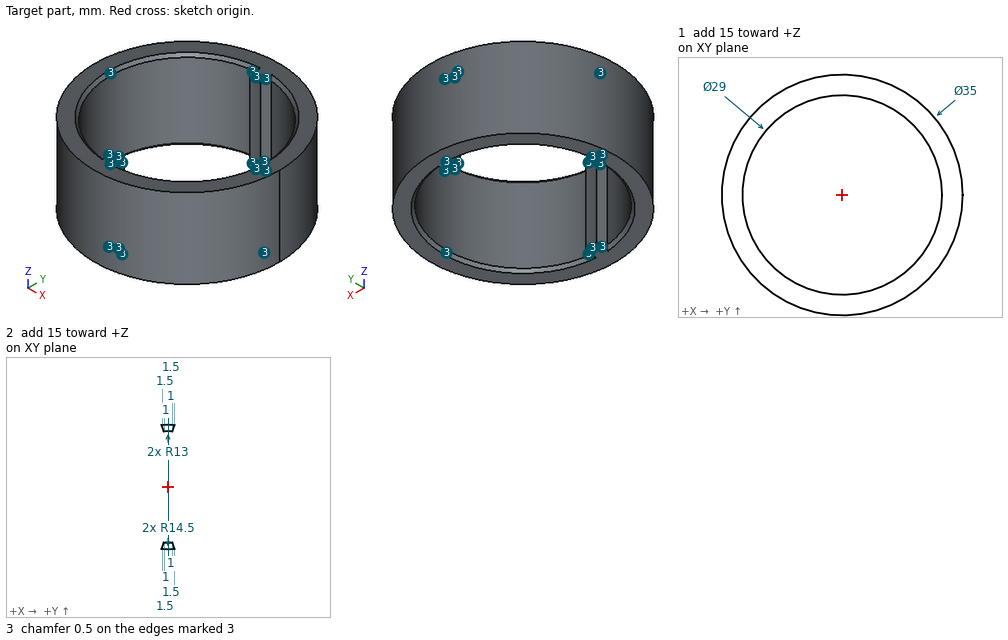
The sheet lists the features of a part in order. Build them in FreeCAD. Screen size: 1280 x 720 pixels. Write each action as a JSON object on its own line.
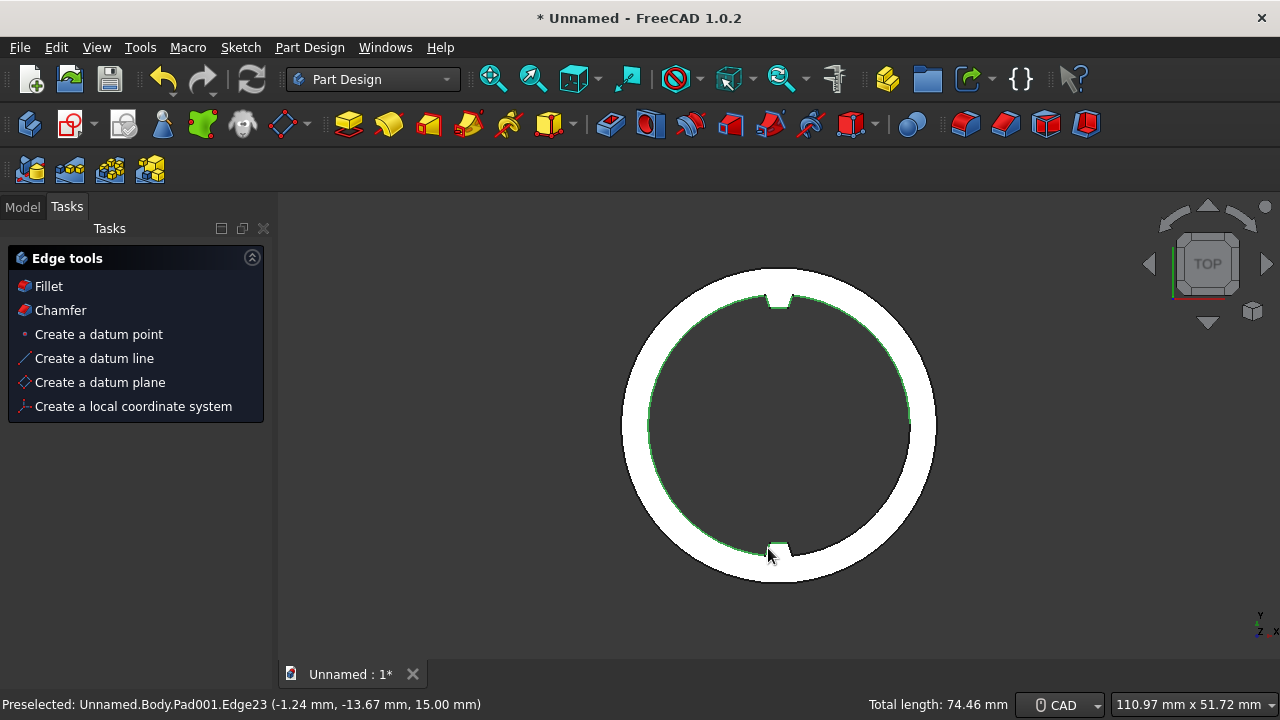
{"action": "left_click", "coordinate": [790, 548], "text": "ctrl"}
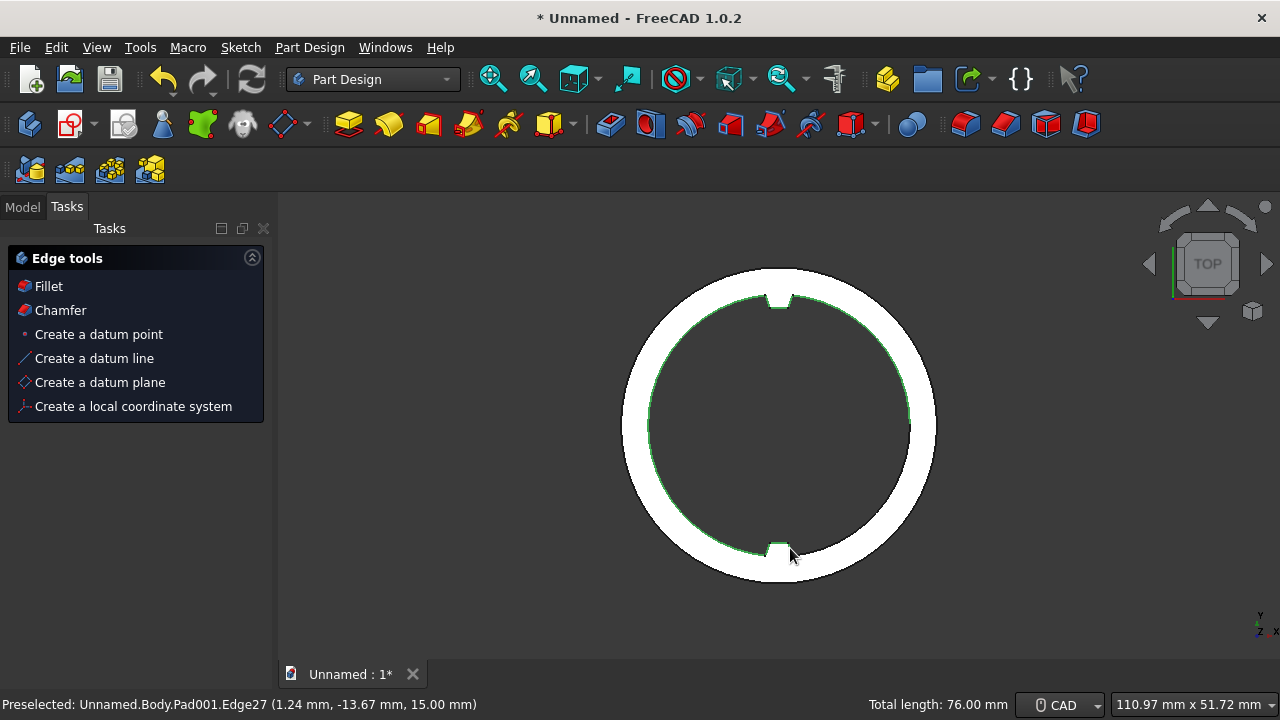
{"action": "key", "text": "1"}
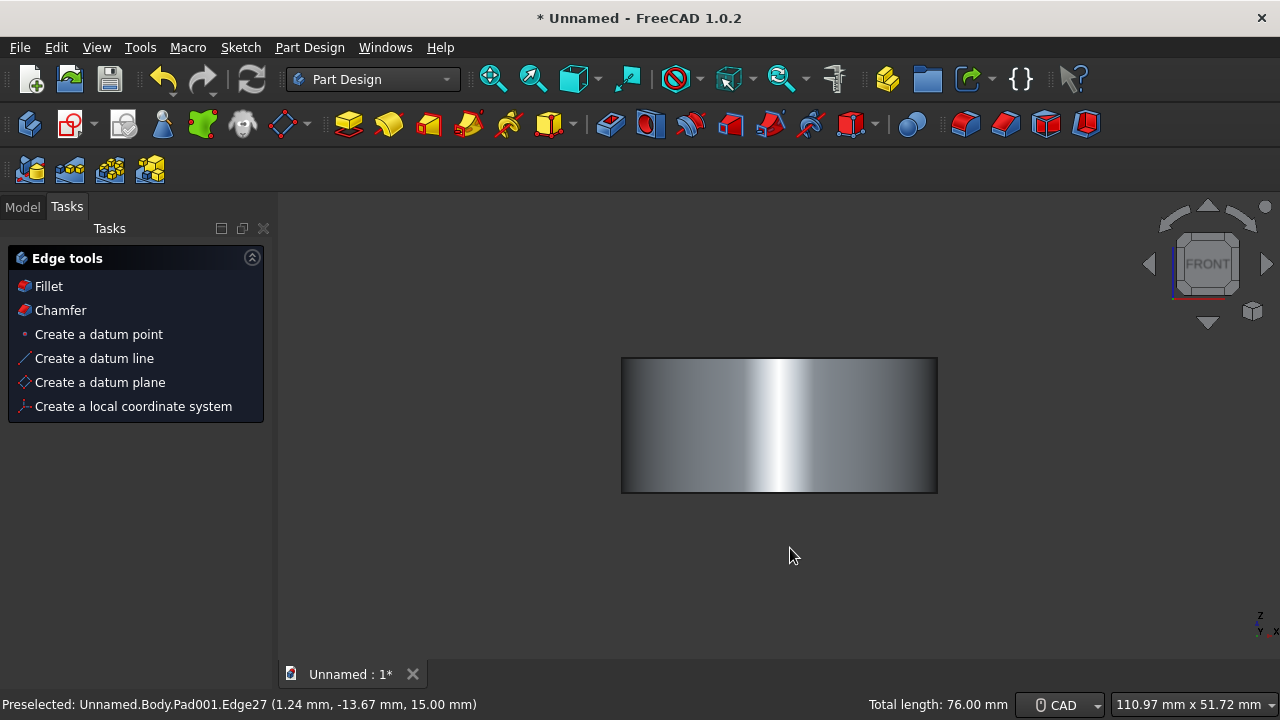
{"action": "left_click", "coordinate": [494, 80]}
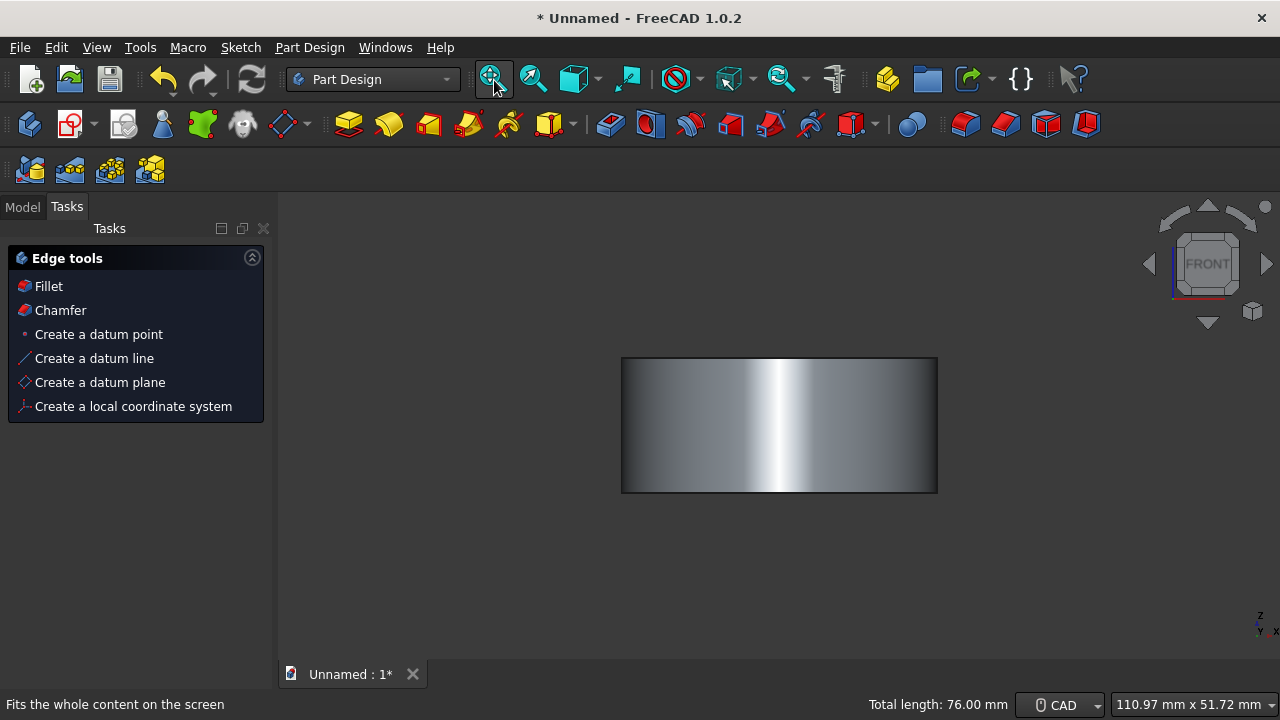
{"action": "key", "text": "3"}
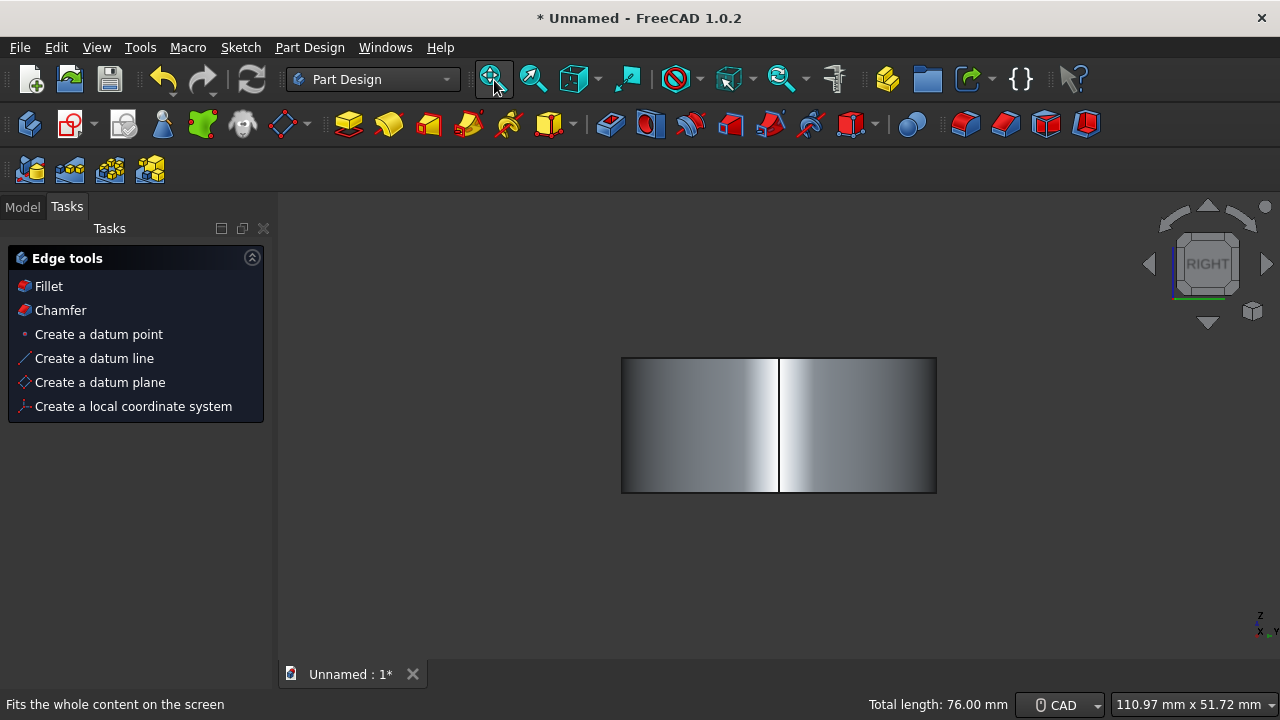
{"action": "left_click", "coordinate": [494, 80]}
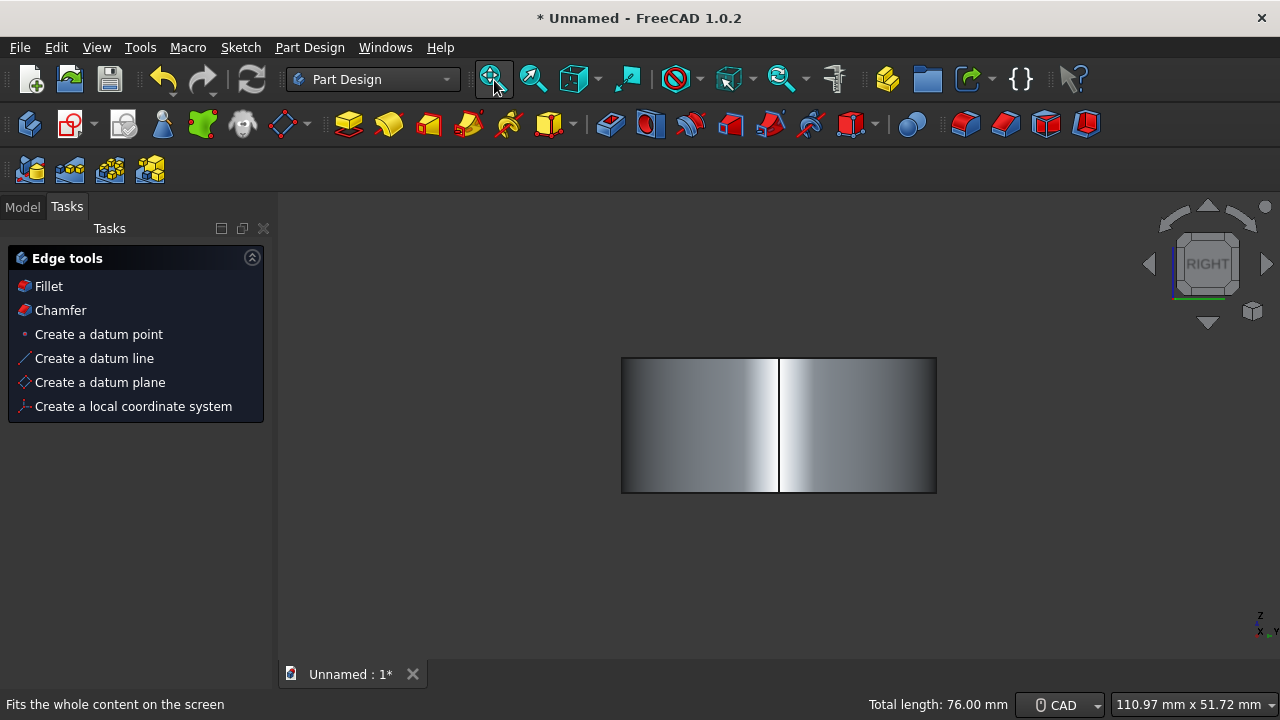
{"action": "key", "text": "5"}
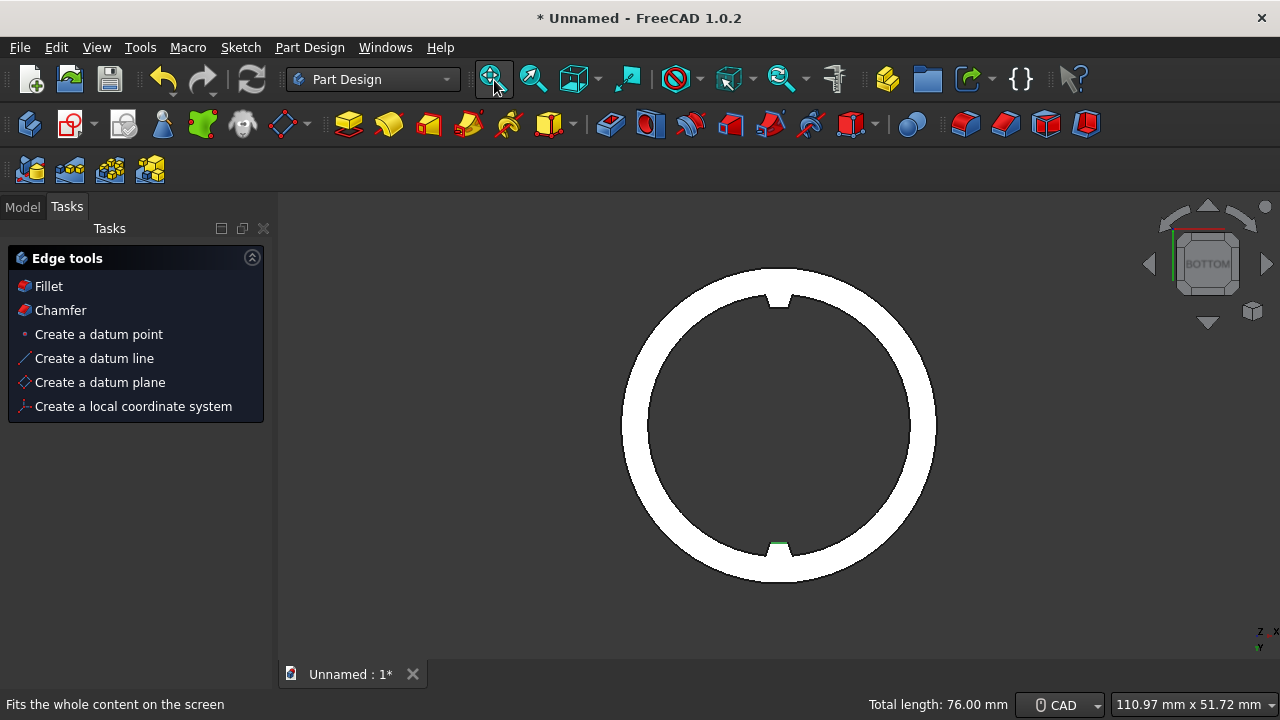
{"action": "left_click", "coordinate": [648, 424], "text": "ctrl"}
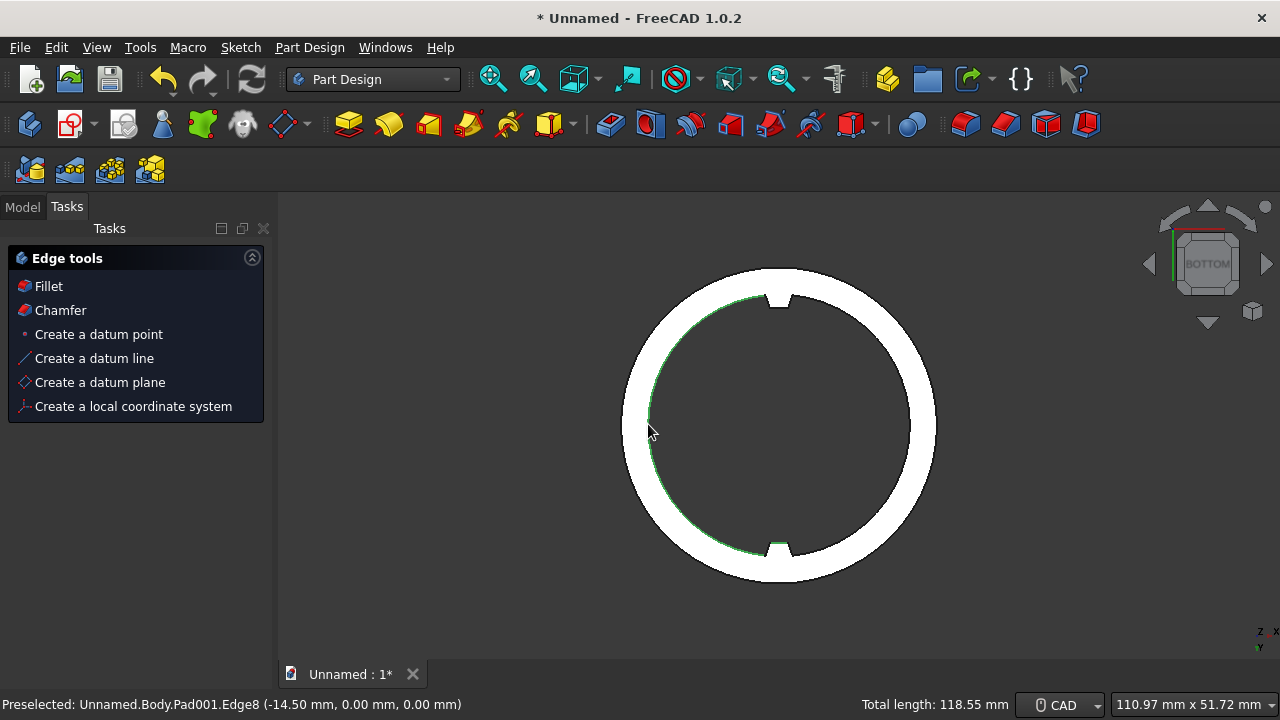
{"action": "left_click", "coordinate": [768, 548], "text": "ctrl"}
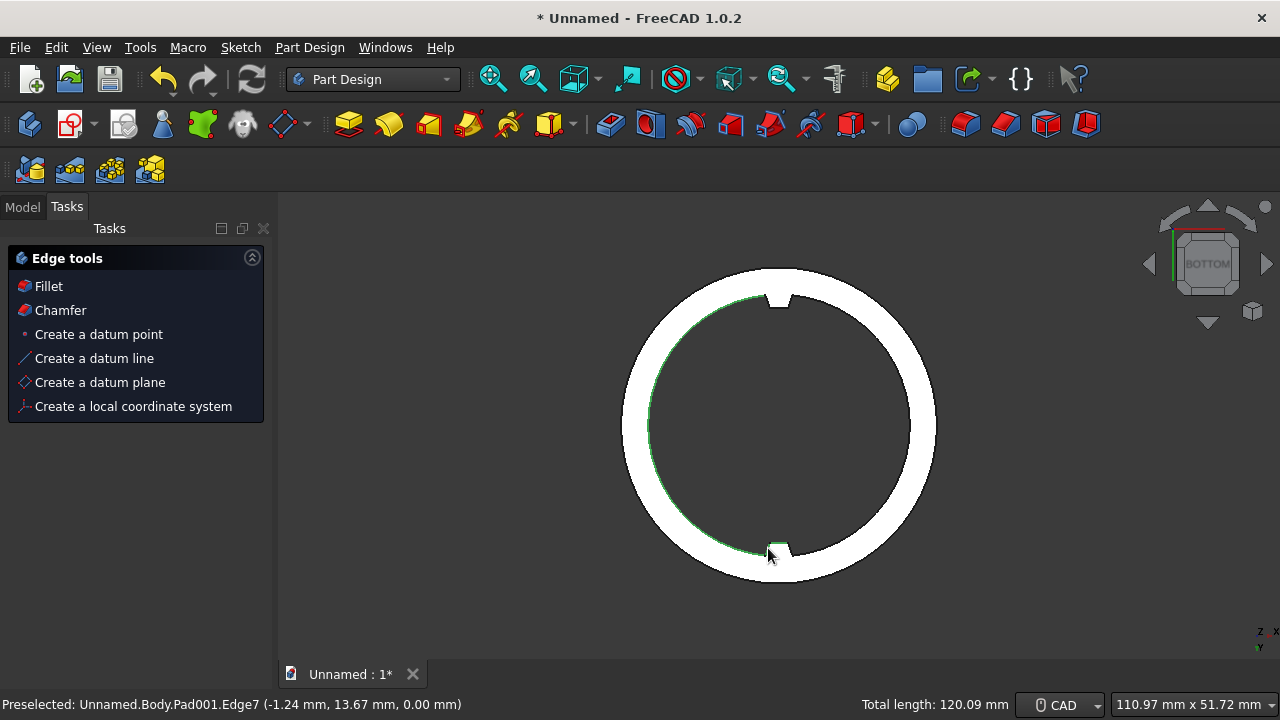
{"action": "left_click", "coordinate": [790, 548], "text": "ctrl"}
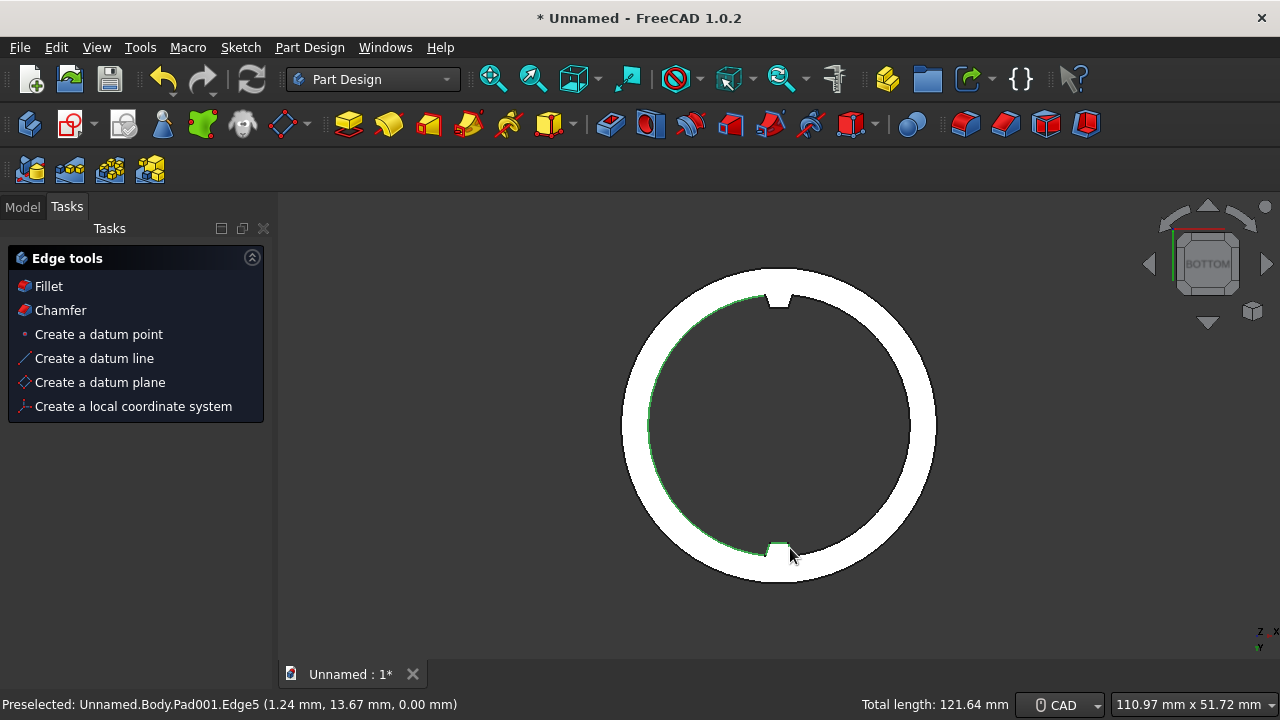
{"action": "left_click", "coordinate": [862, 525], "text": "ctrl"}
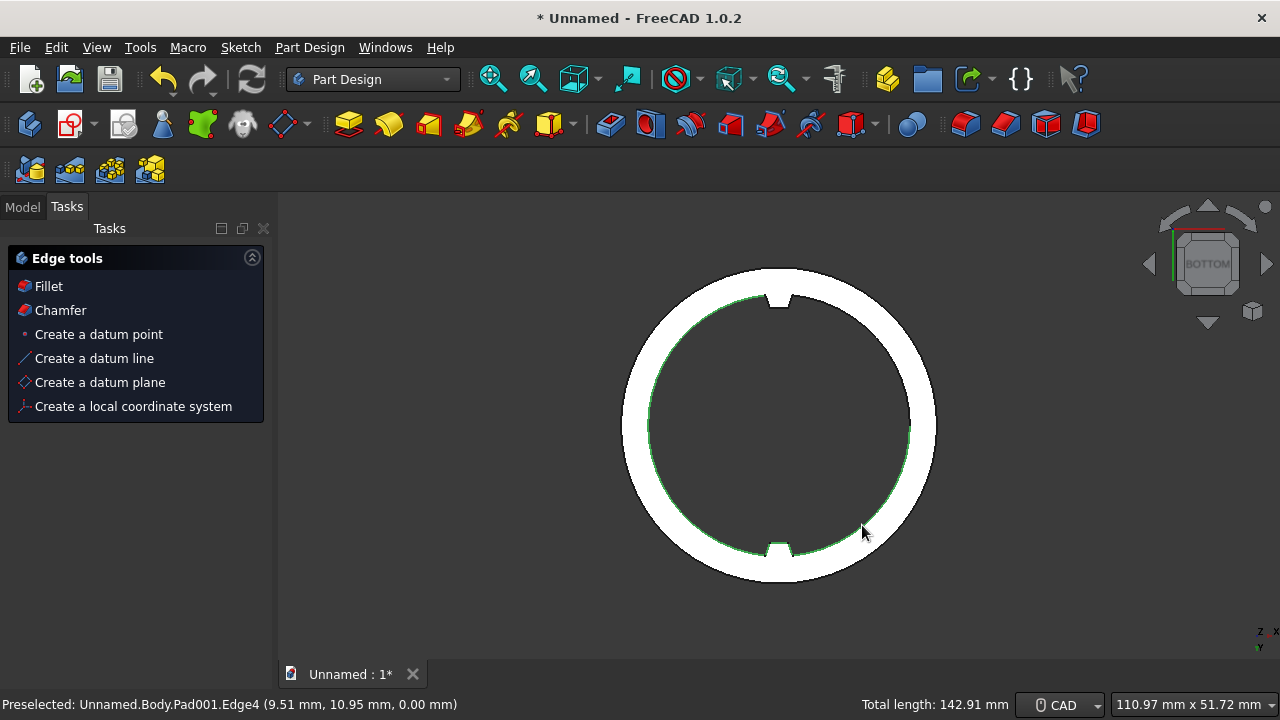
{"action": "left_click", "coordinate": [790, 301], "text": "ctrl"}